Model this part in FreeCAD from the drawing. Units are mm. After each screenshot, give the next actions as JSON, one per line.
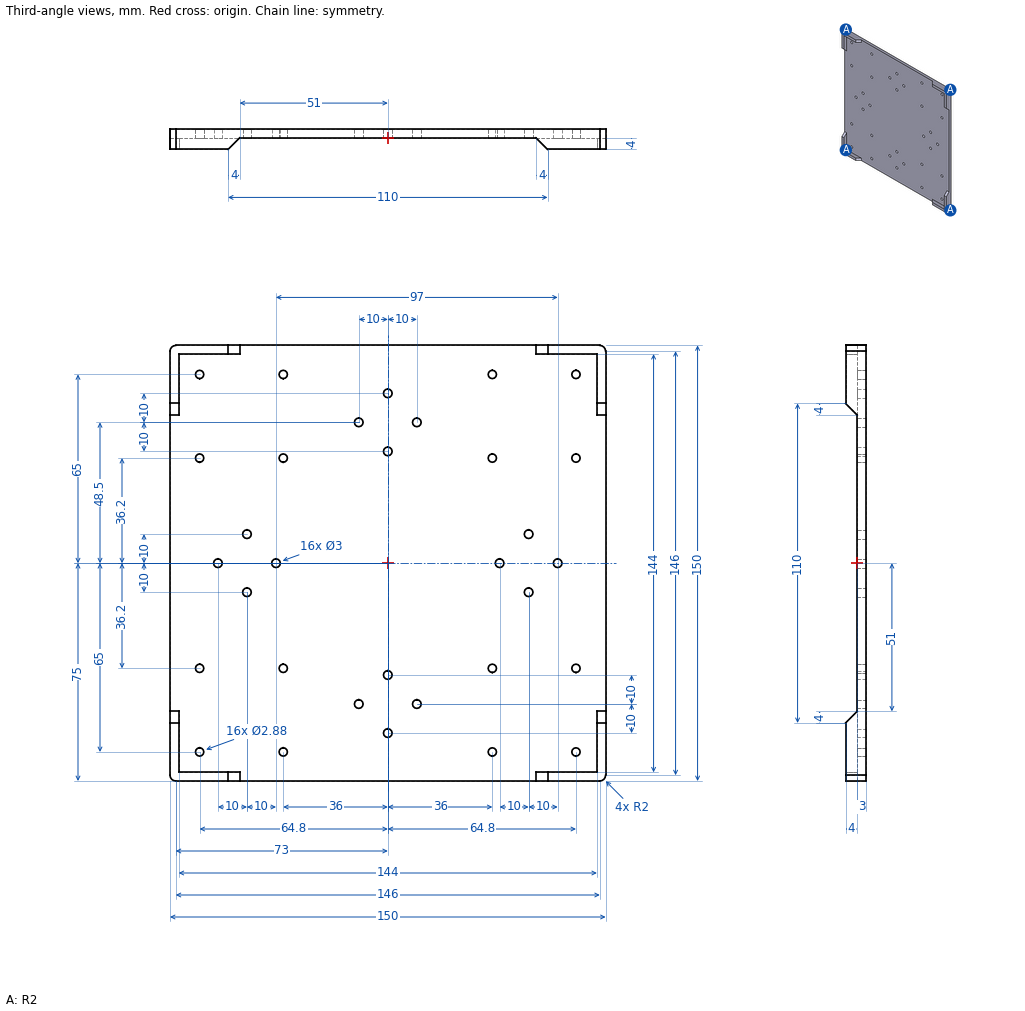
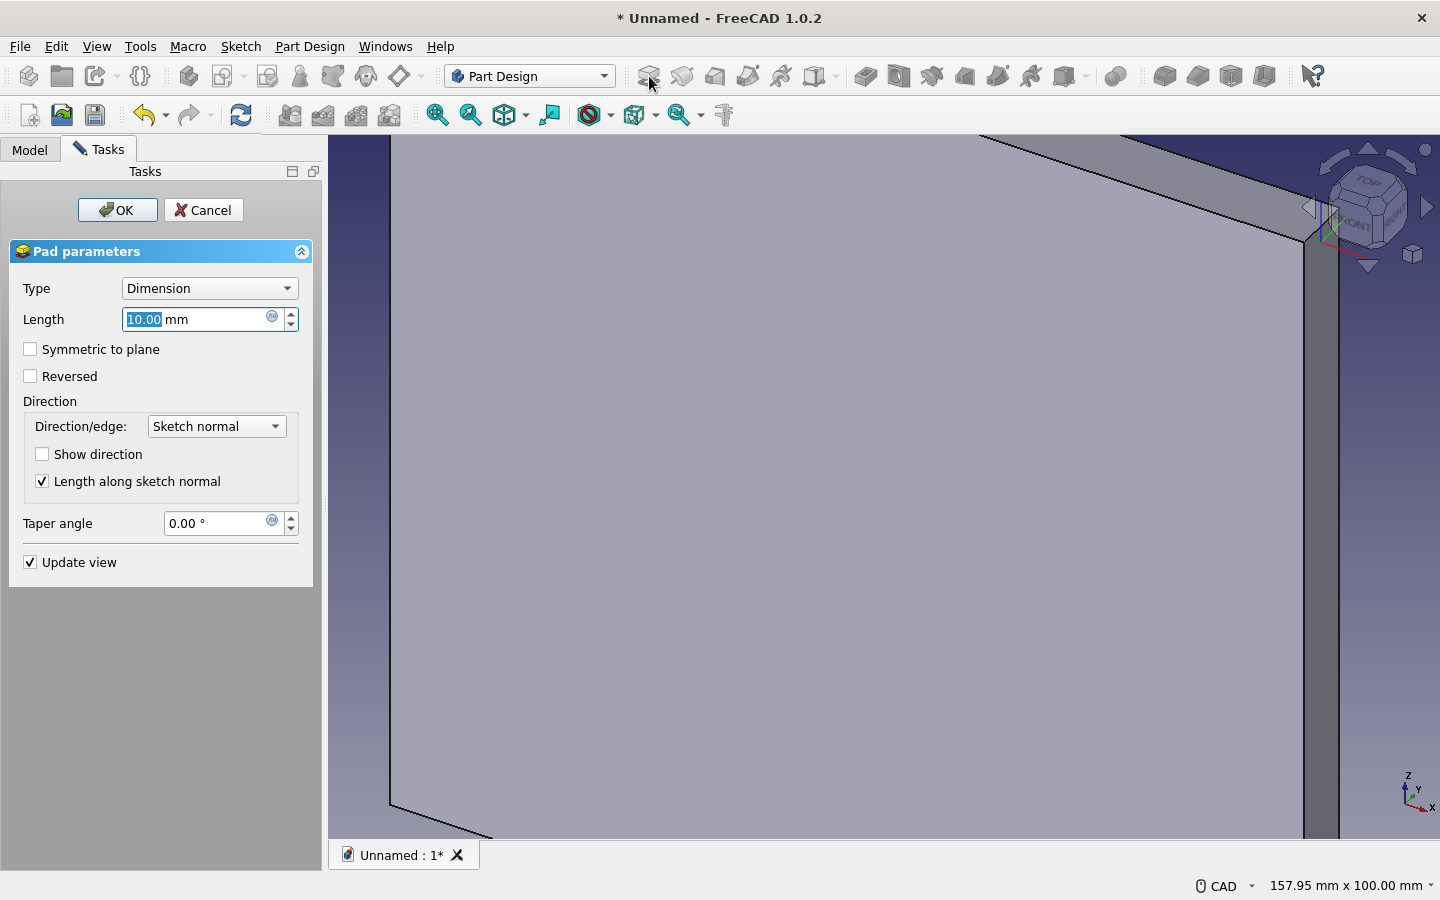
{"action": "type", "text": "3"}
{"action": "key", "text": "Tab"}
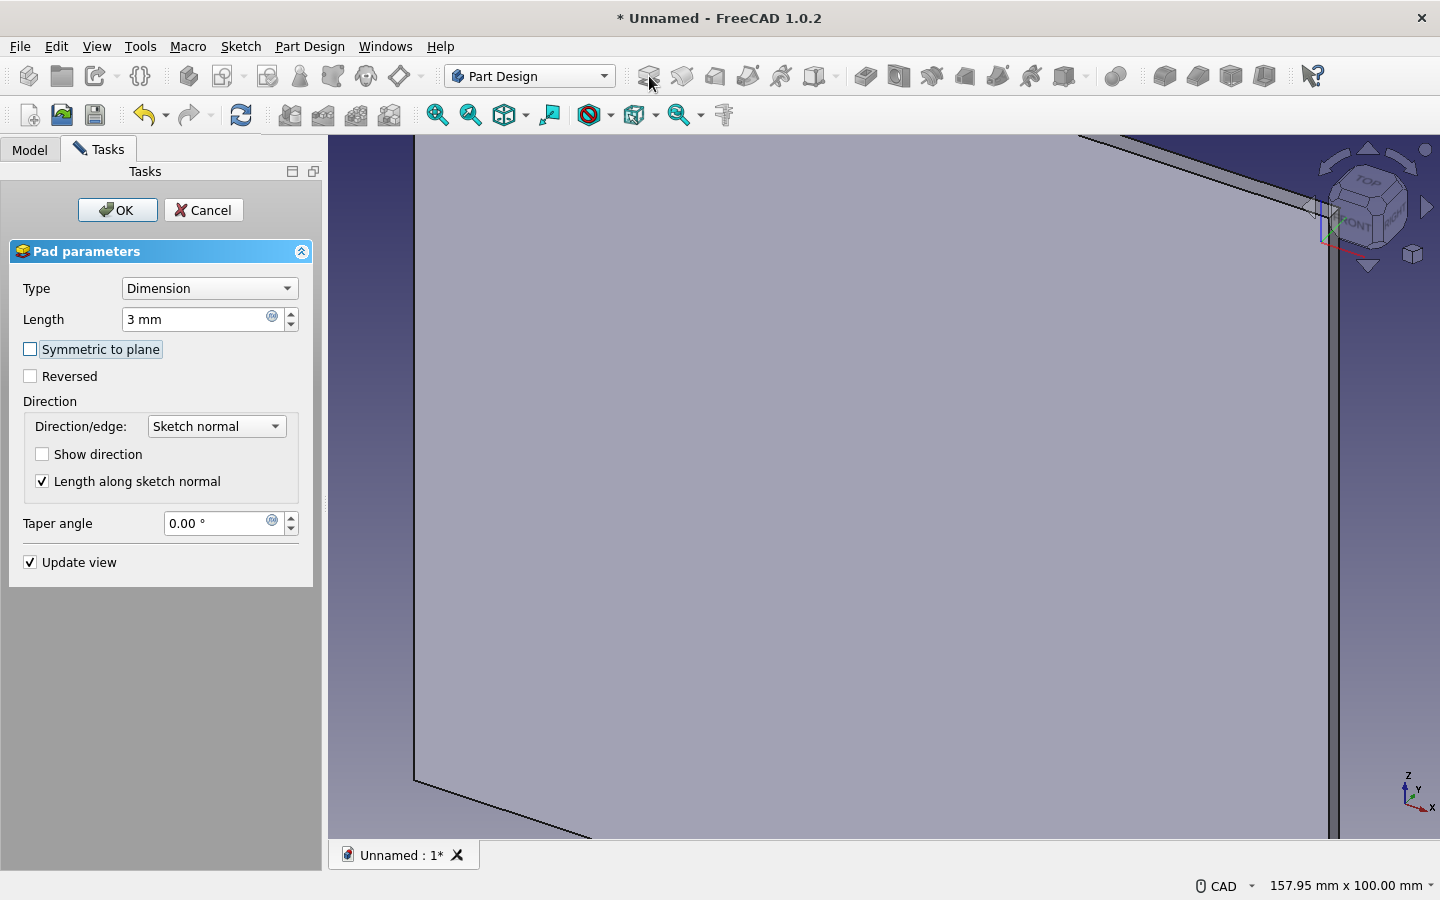
{"action": "left_click", "coordinate": [31, 376]}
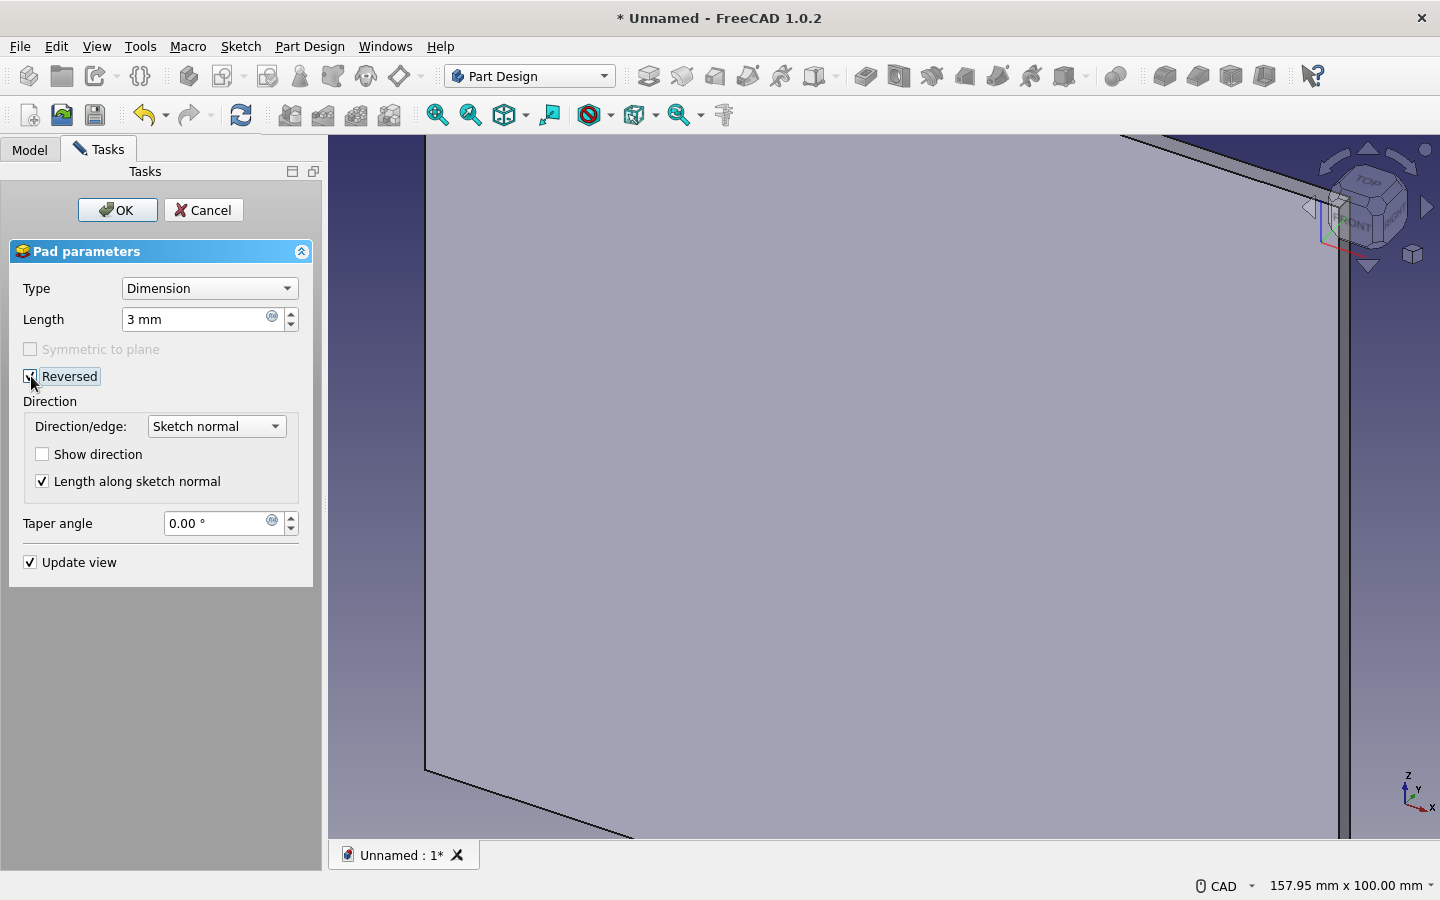
{"action": "left_click", "coordinate": [118, 210]}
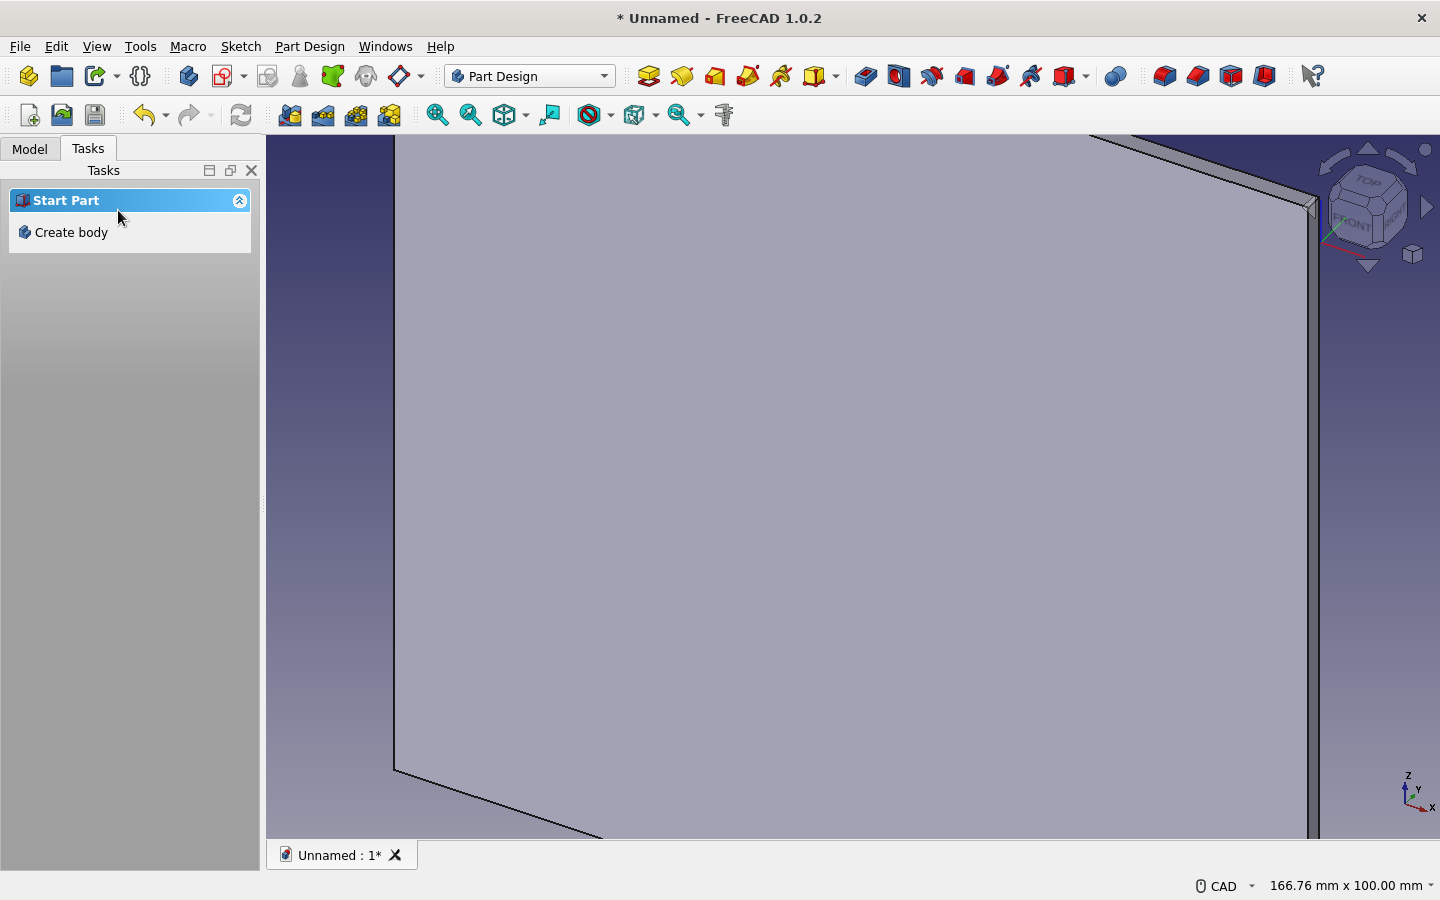
{"action": "key", "text": "v f"}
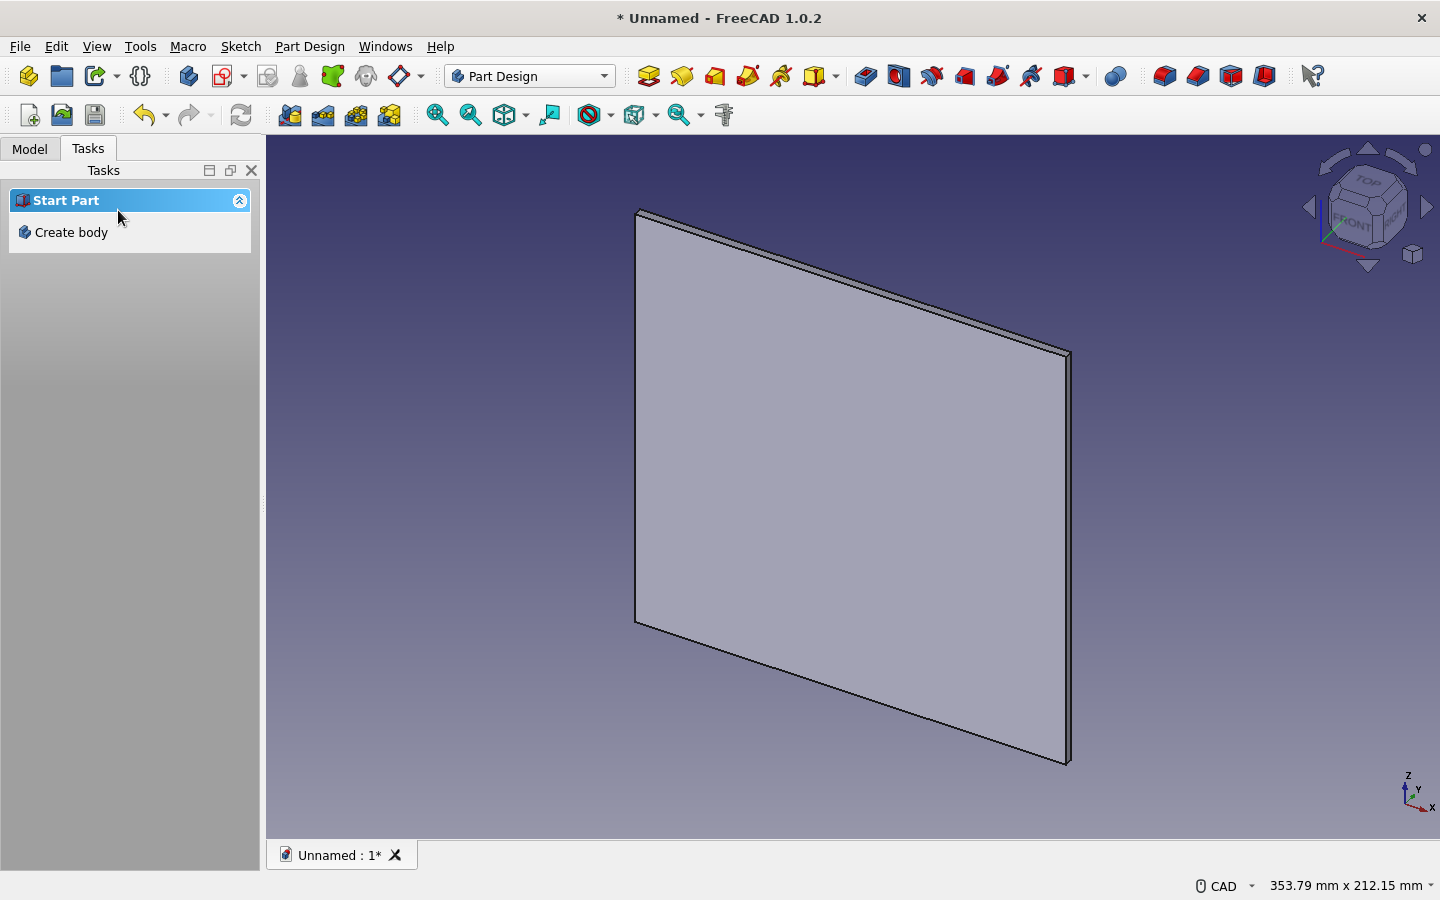
{"action": "key", "text": "4"}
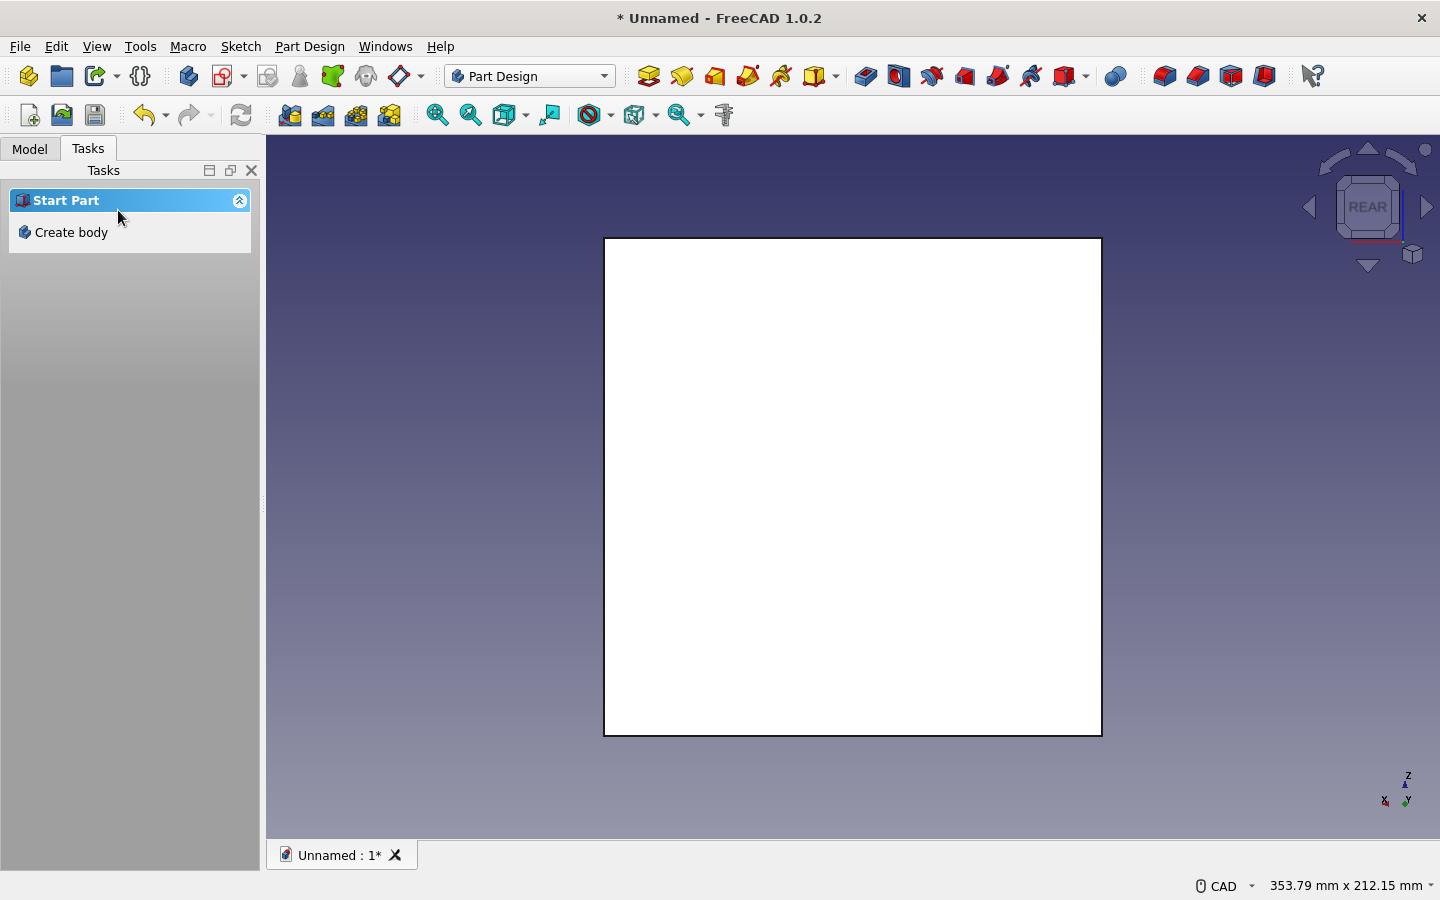
{"action": "left_click", "coordinate": [853, 486]}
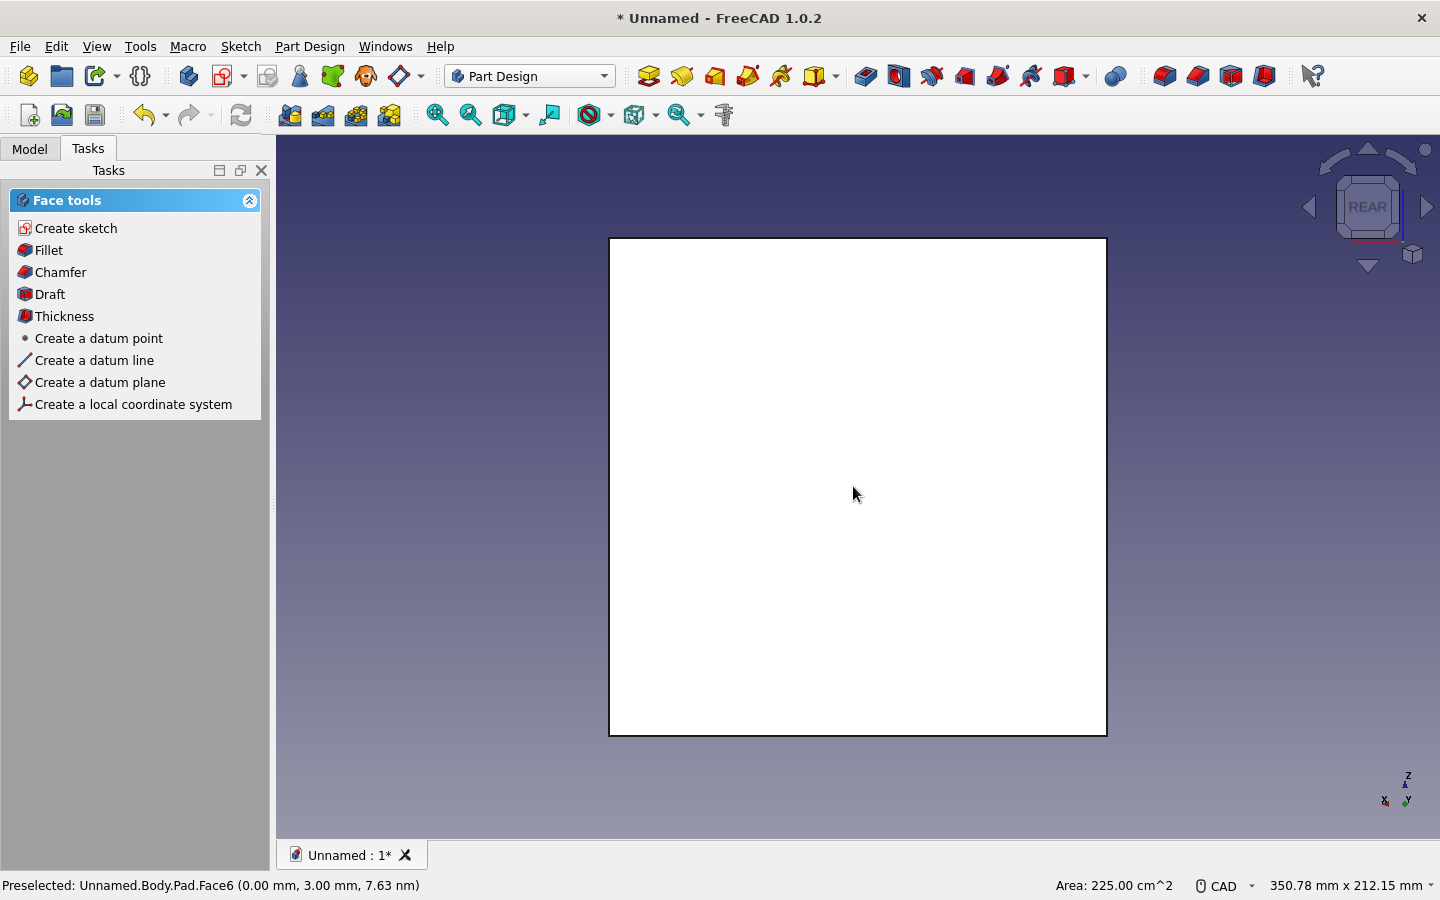
{"action": "left_click", "coordinate": [222, 76]}